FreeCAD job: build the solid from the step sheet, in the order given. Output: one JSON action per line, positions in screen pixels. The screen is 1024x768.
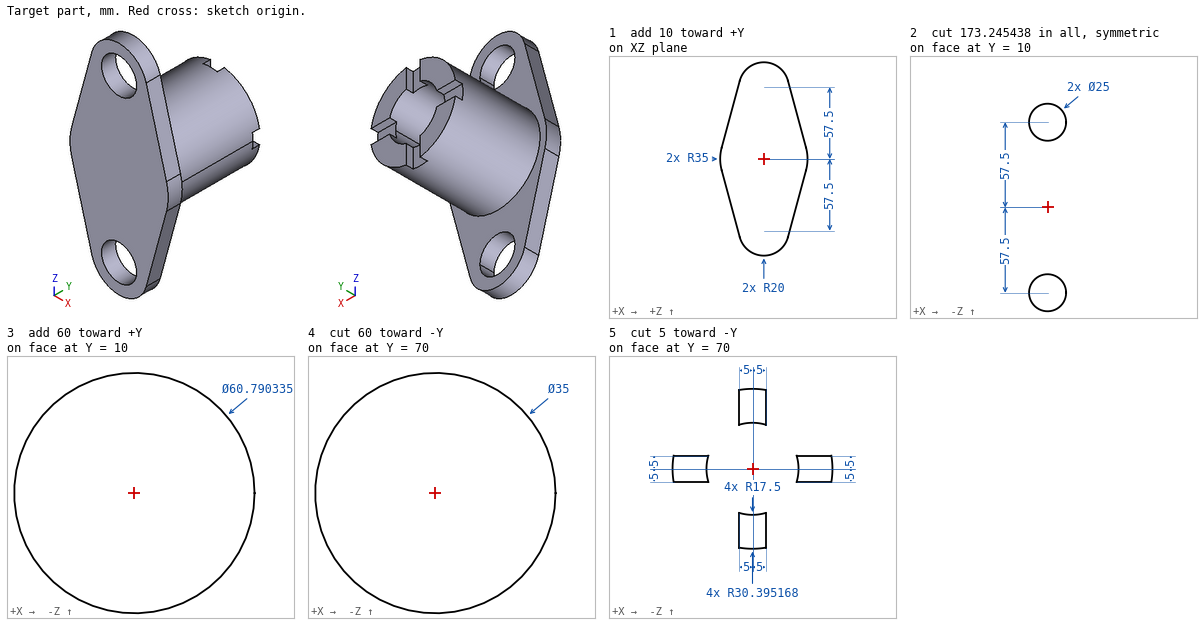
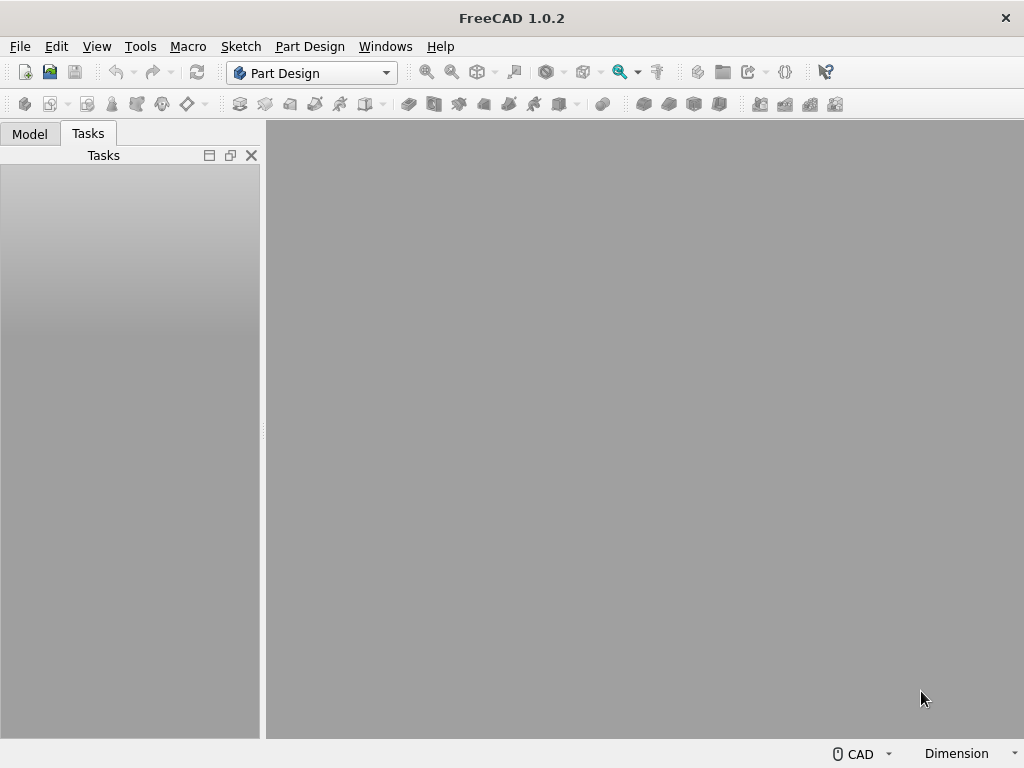
{"action": "left_click", "coordinate": [25, 72]}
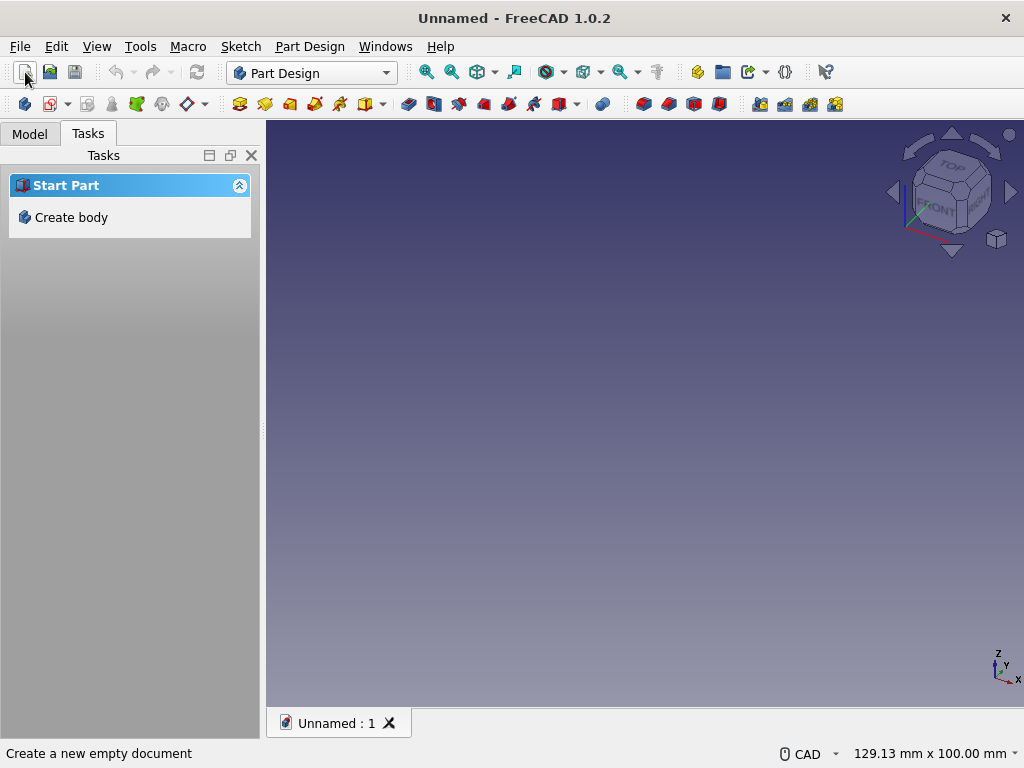
{"action": "left_click", "coordinate": [50, 104]}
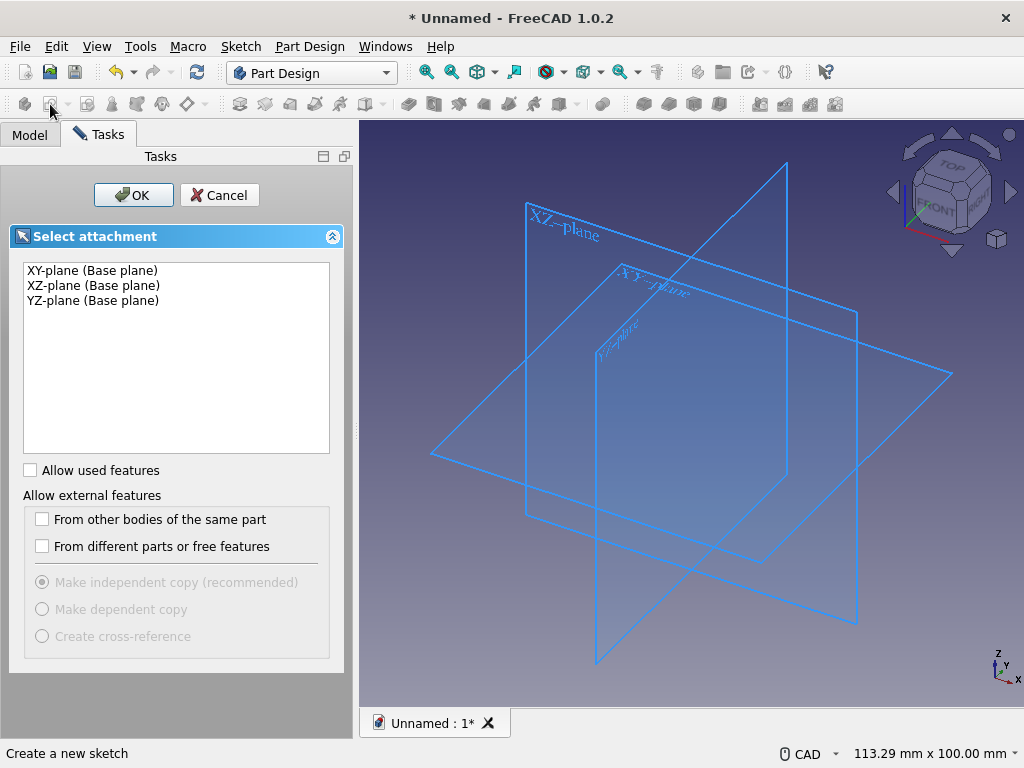
{"action": "left_click", "coordinate": [84, 286]}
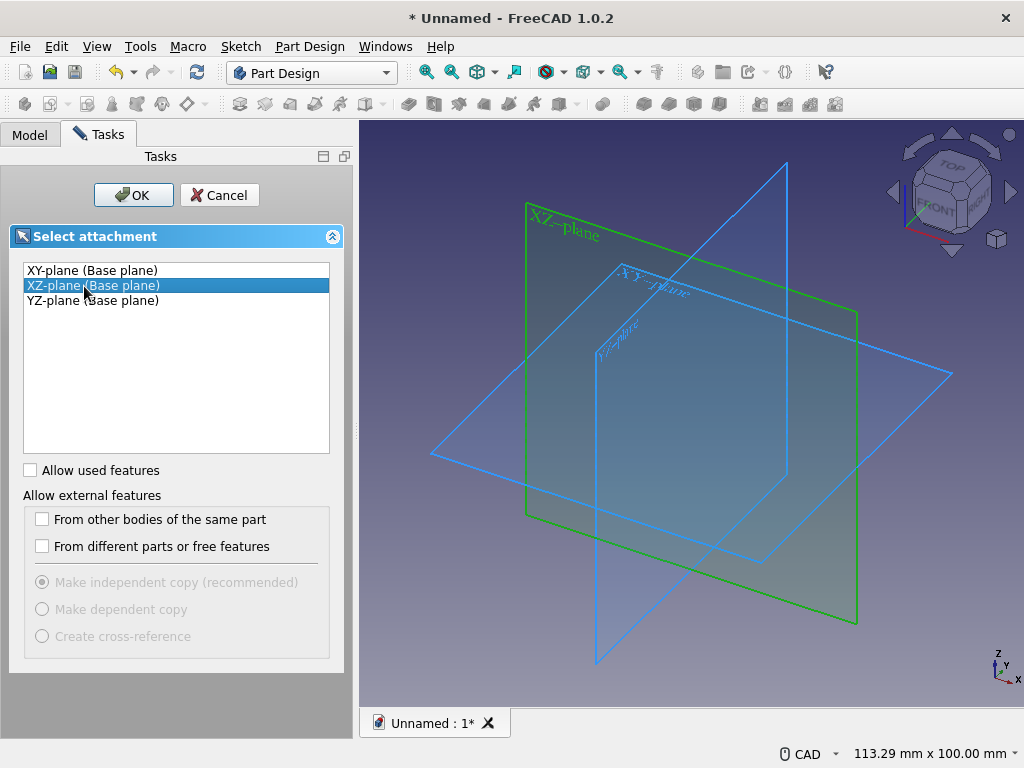
{"action": "left_click", "coordinate": [134, 195]}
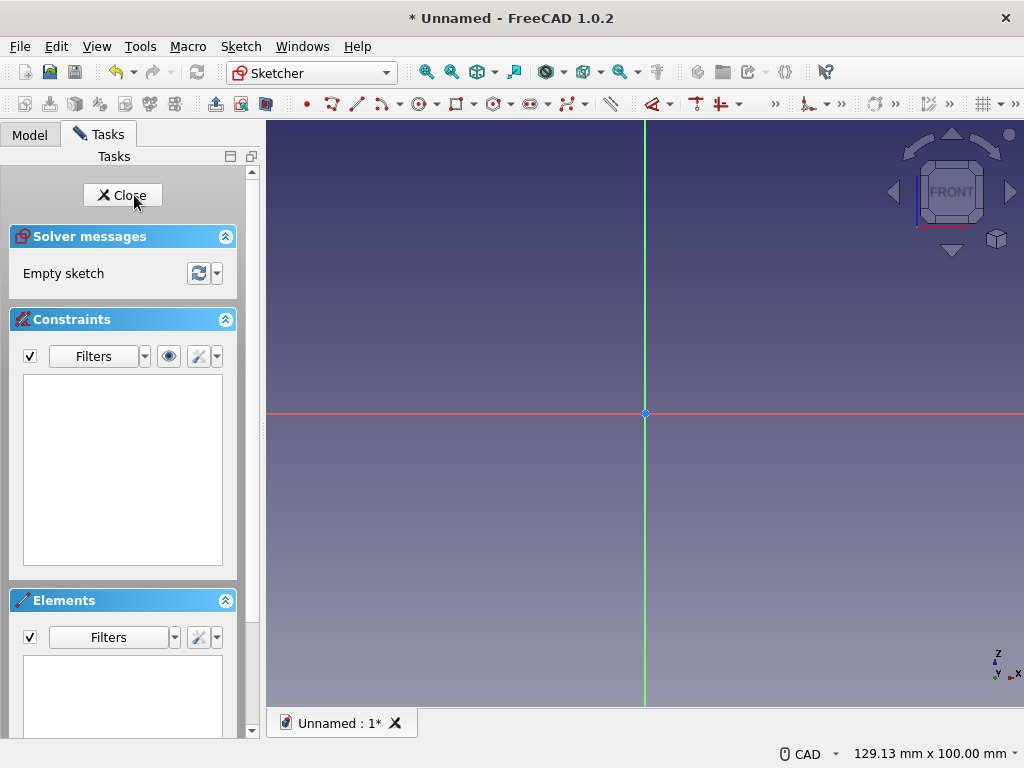
{"action": "scroll", "coordinate": [521, 414], "scroll_direction": "down", "scroll_amount": 4}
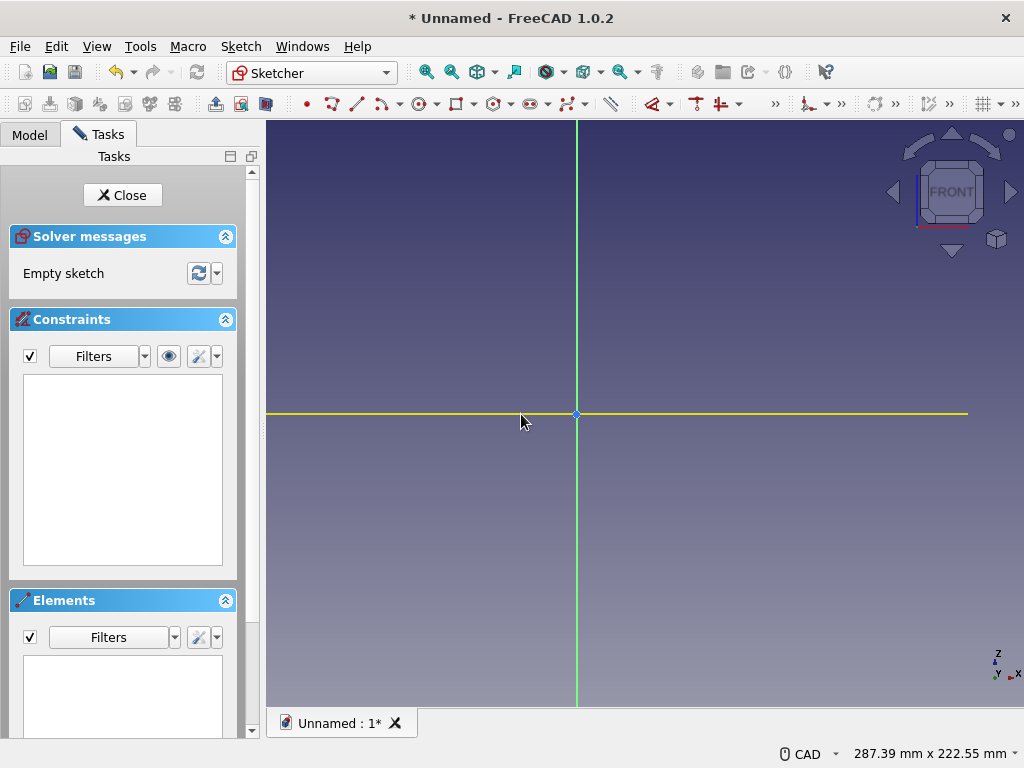
{"action": "key", "text": "g l"}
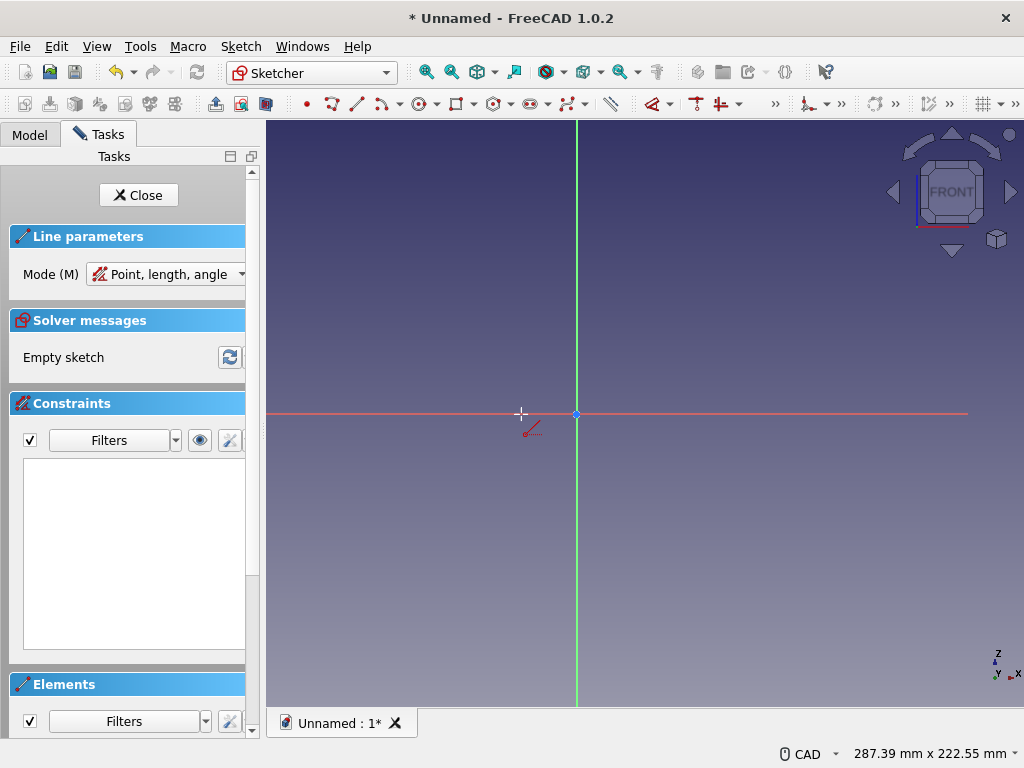
{"action": "left_click", "coordinate": [628, 249]}
{"action": "left_click", "coordinate": [666, 390]}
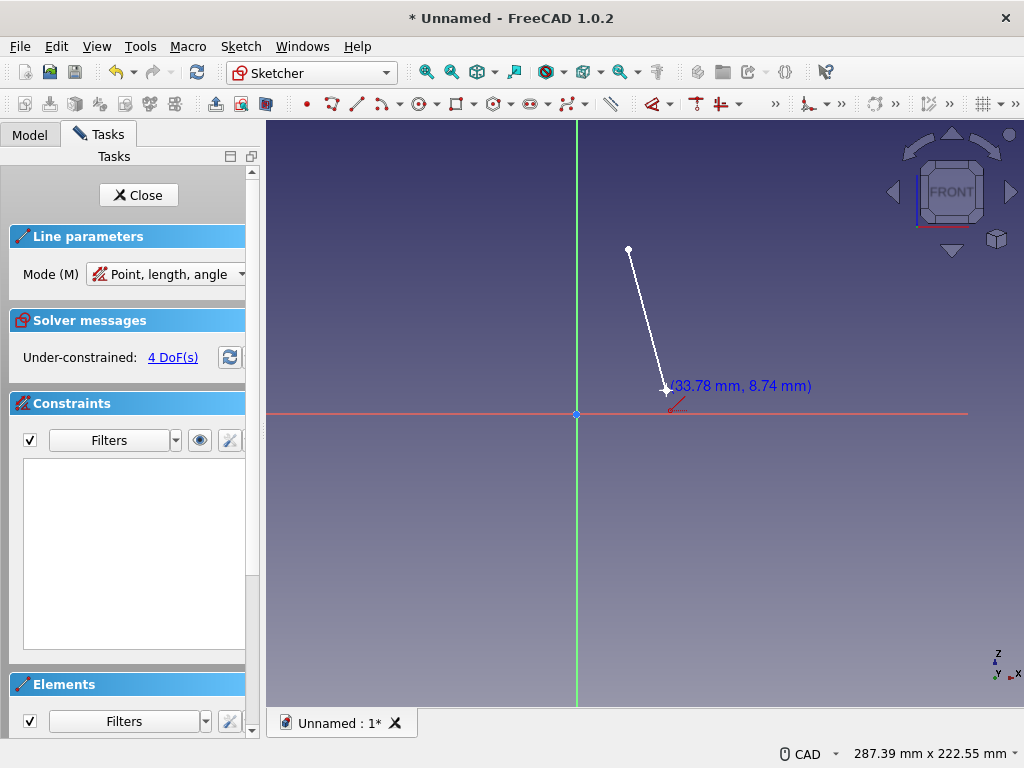
{"action": "left_click", "coordinate": [666, 438]}
{"action": "left_click", "coordinate": [628, 579]}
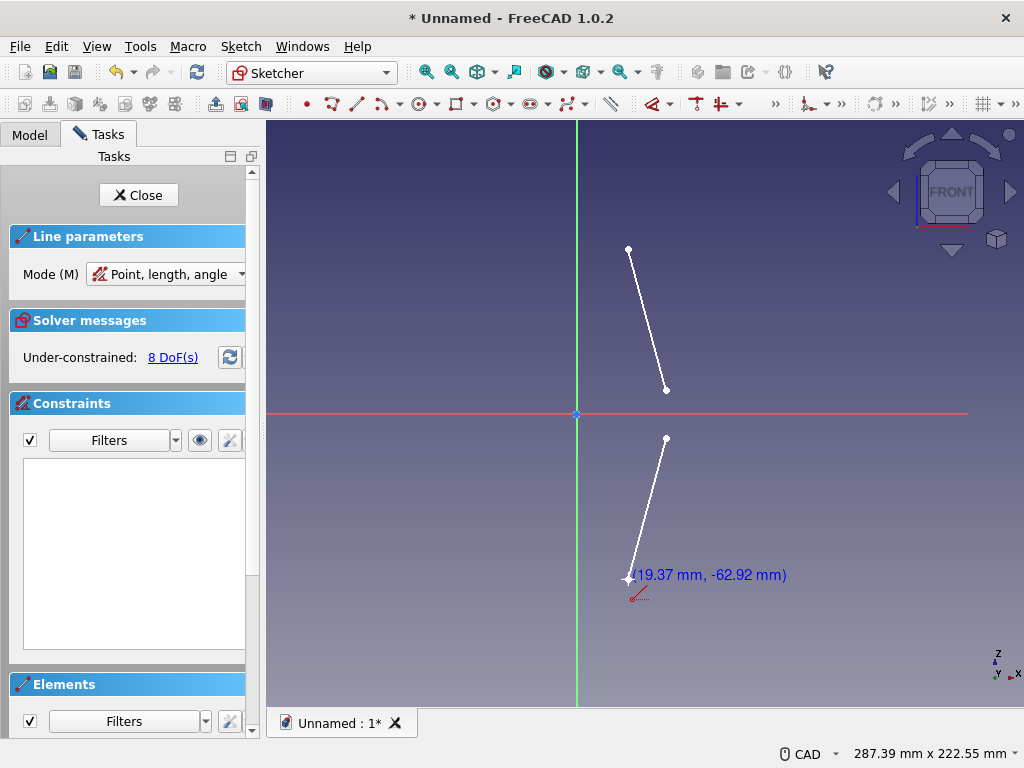
{"action": "left_click", "coordinate": [526, 579]}
{"action": "left_click", "coordinate": [488, 438]}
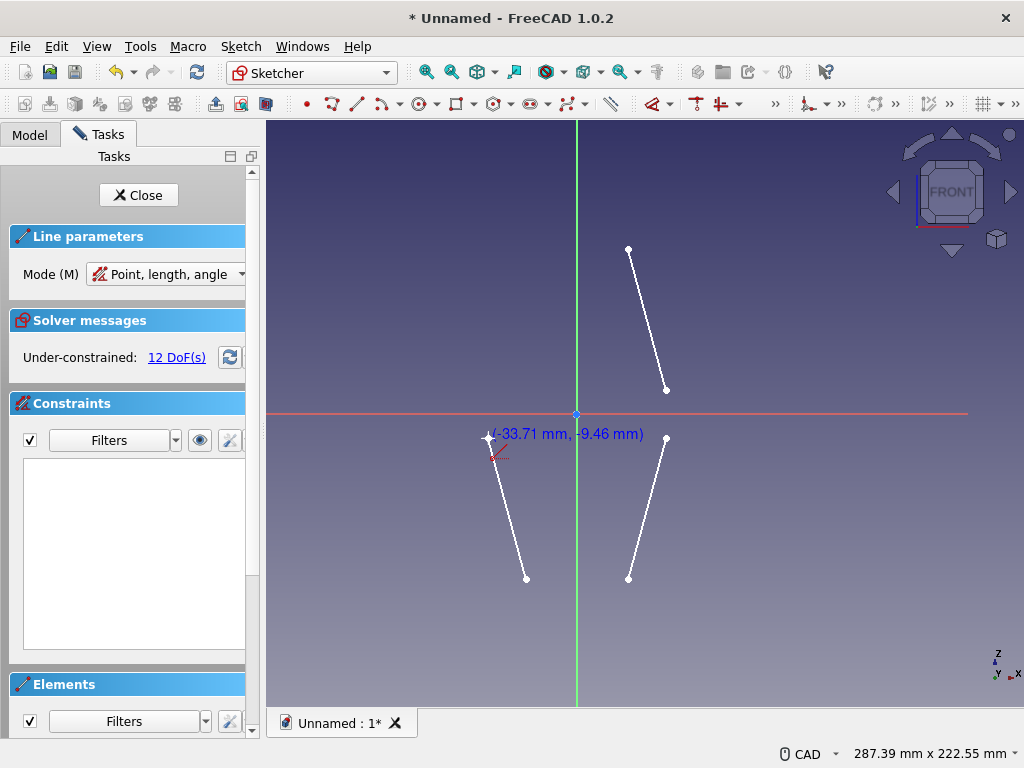
{"action": "left_click", "coordinate": [488, 390]}
{"action": "left_click", "coordinate": [526, 249]}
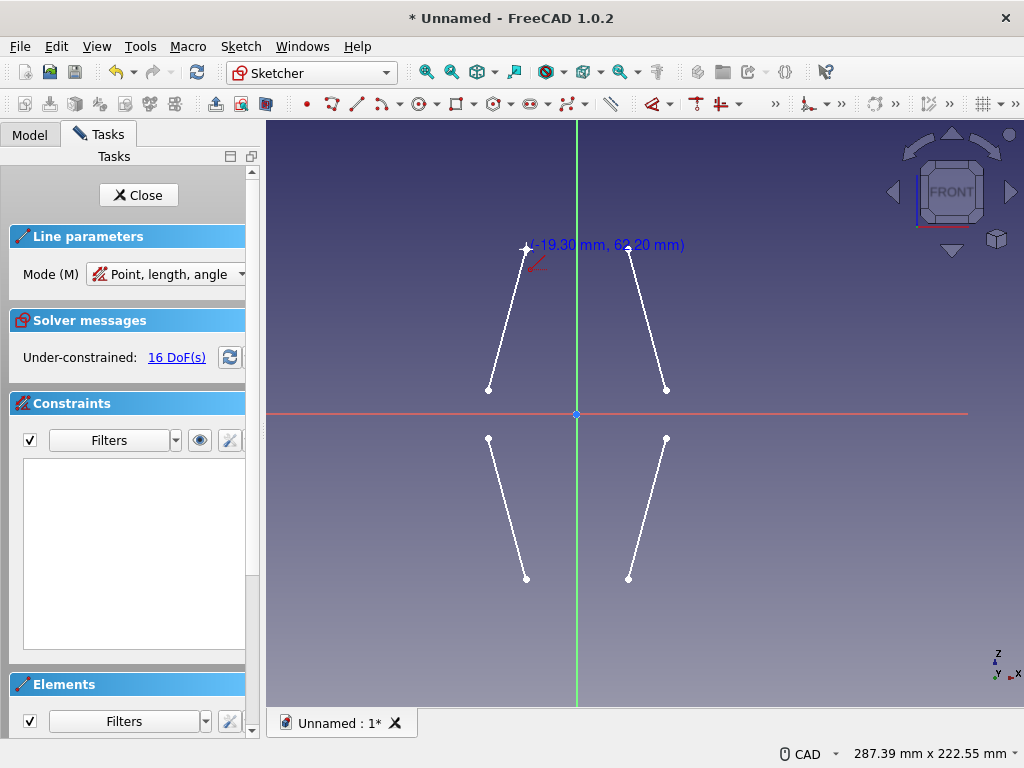
{"action": "key", "text": "g 3 a"}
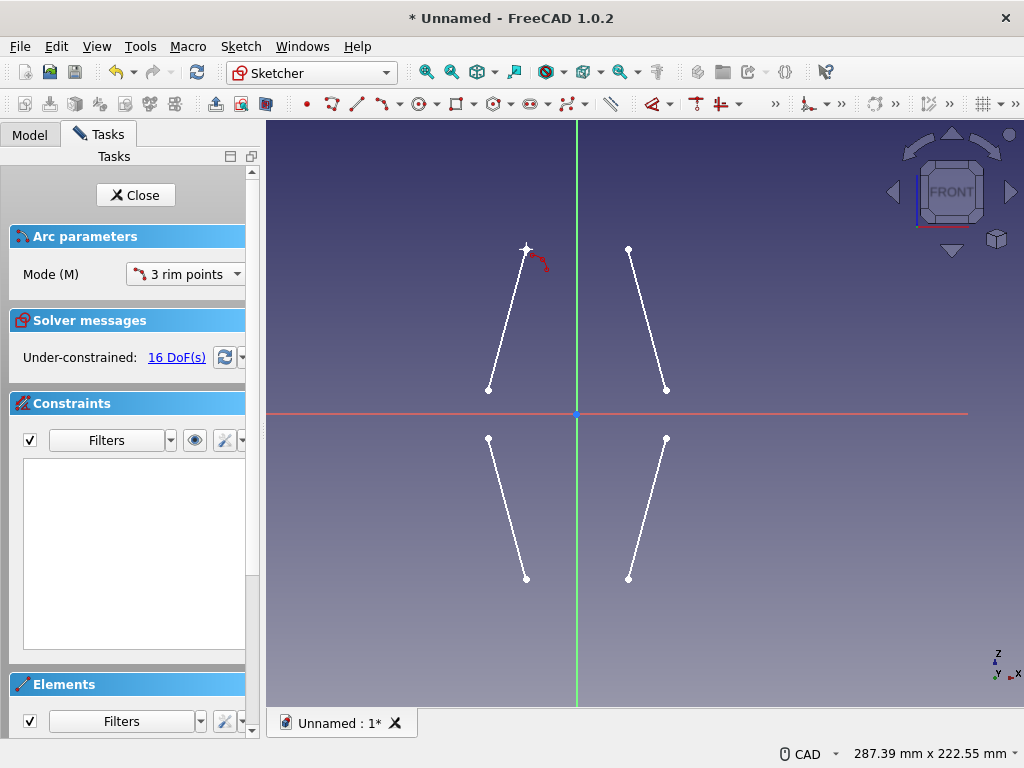
{"action": "left_click", "coordinate": [666, 391]}
{"action": "left_click", "coordinate": [666, 439]}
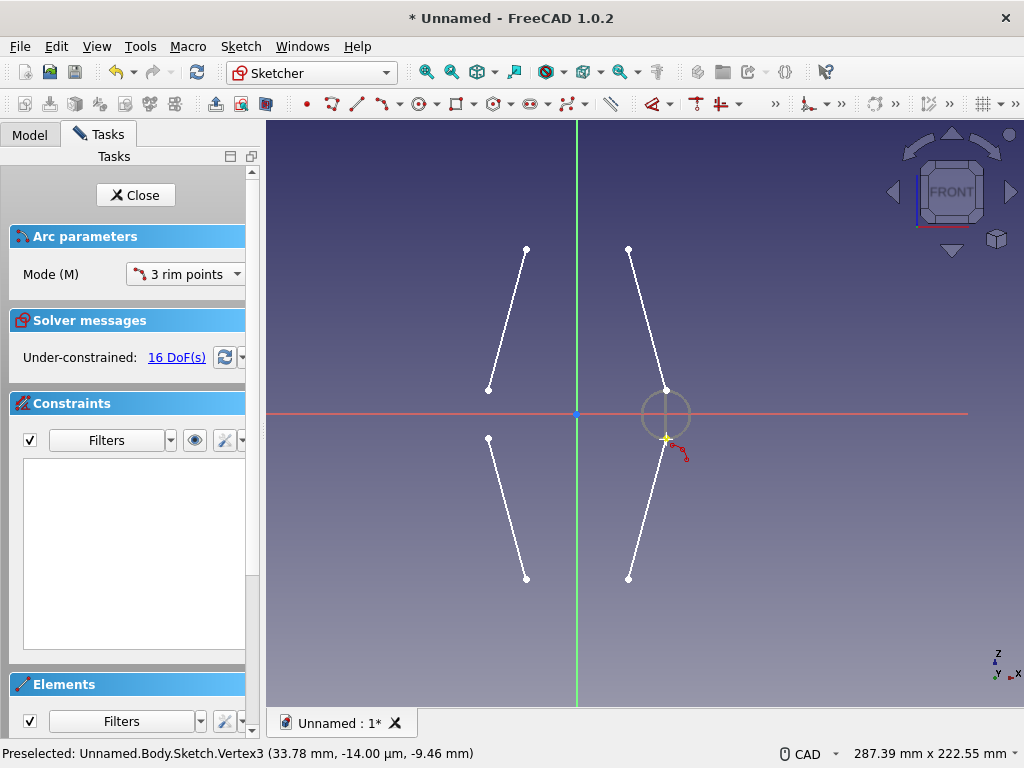
{"action": "scroll", "coordinate": [669, 419], "scroll_direction": "up", "scroll_amount": 9}